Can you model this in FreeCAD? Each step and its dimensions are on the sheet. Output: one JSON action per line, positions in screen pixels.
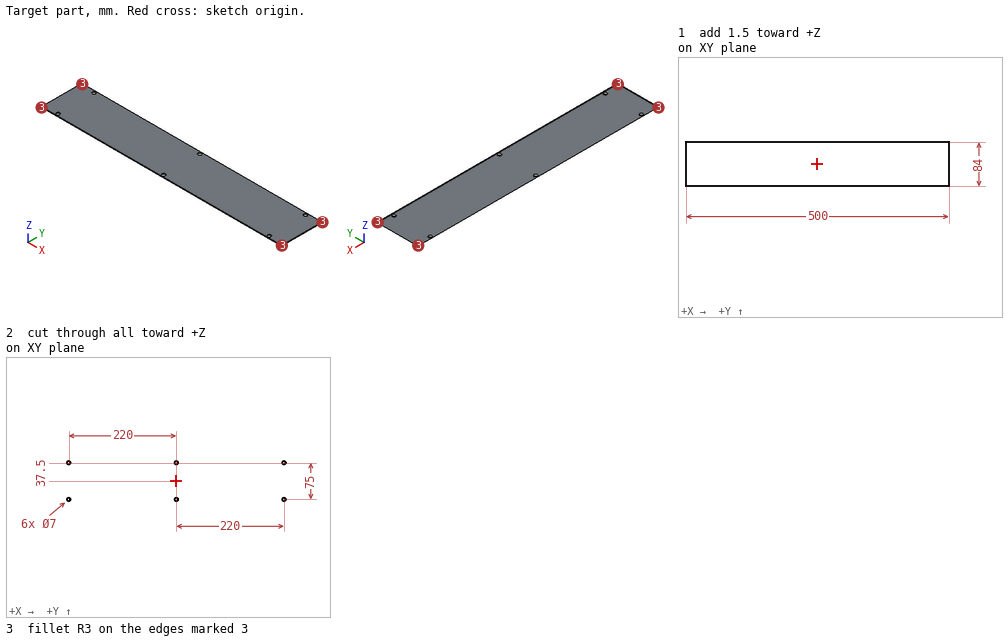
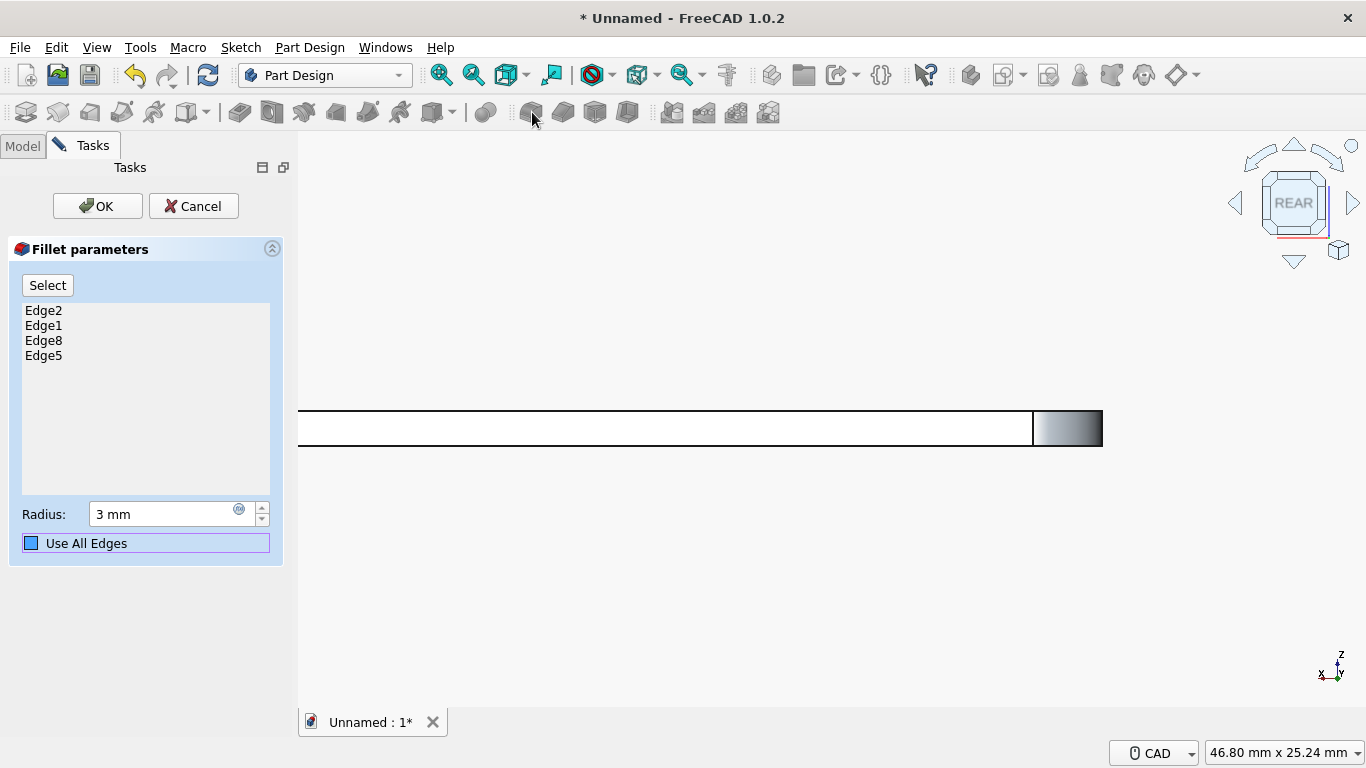
{"action": "left_click", "coordinate": [98, 206]}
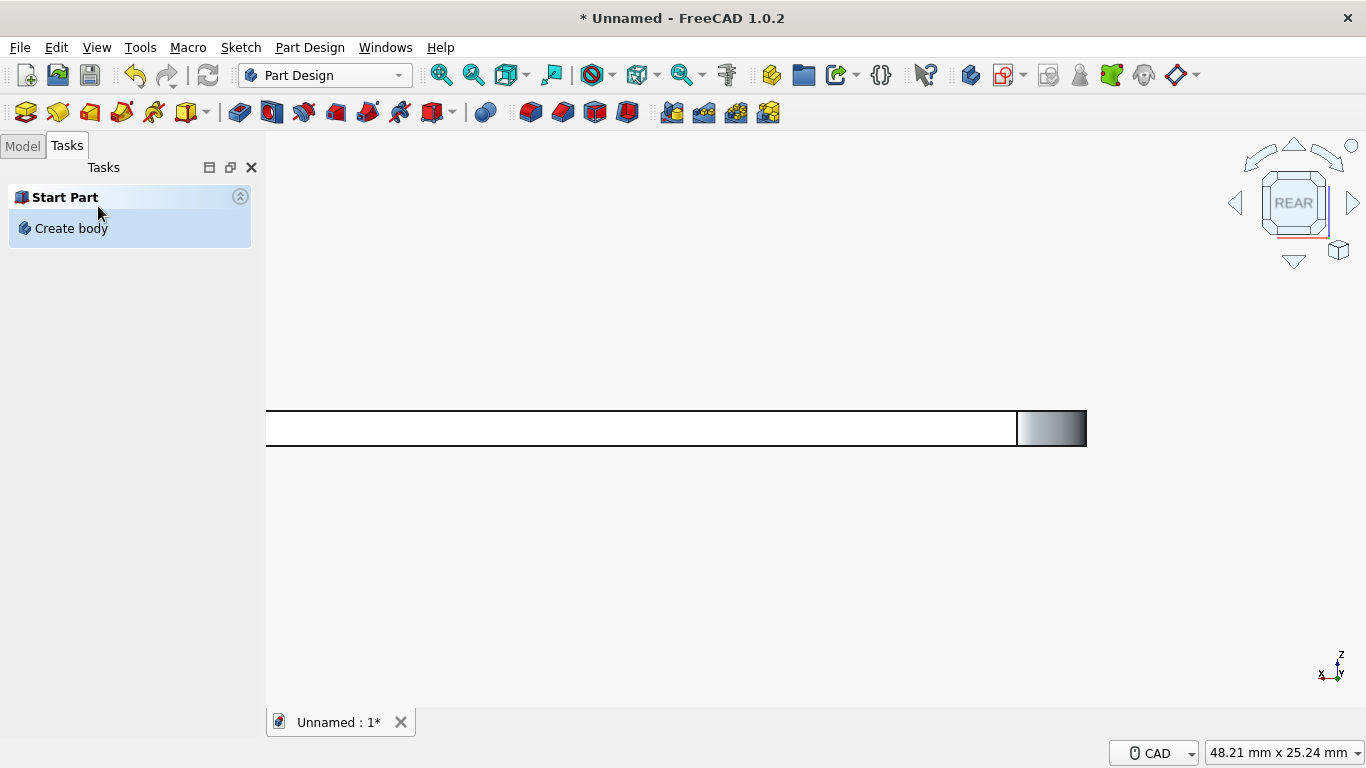
{"action": "key", "text": "0"}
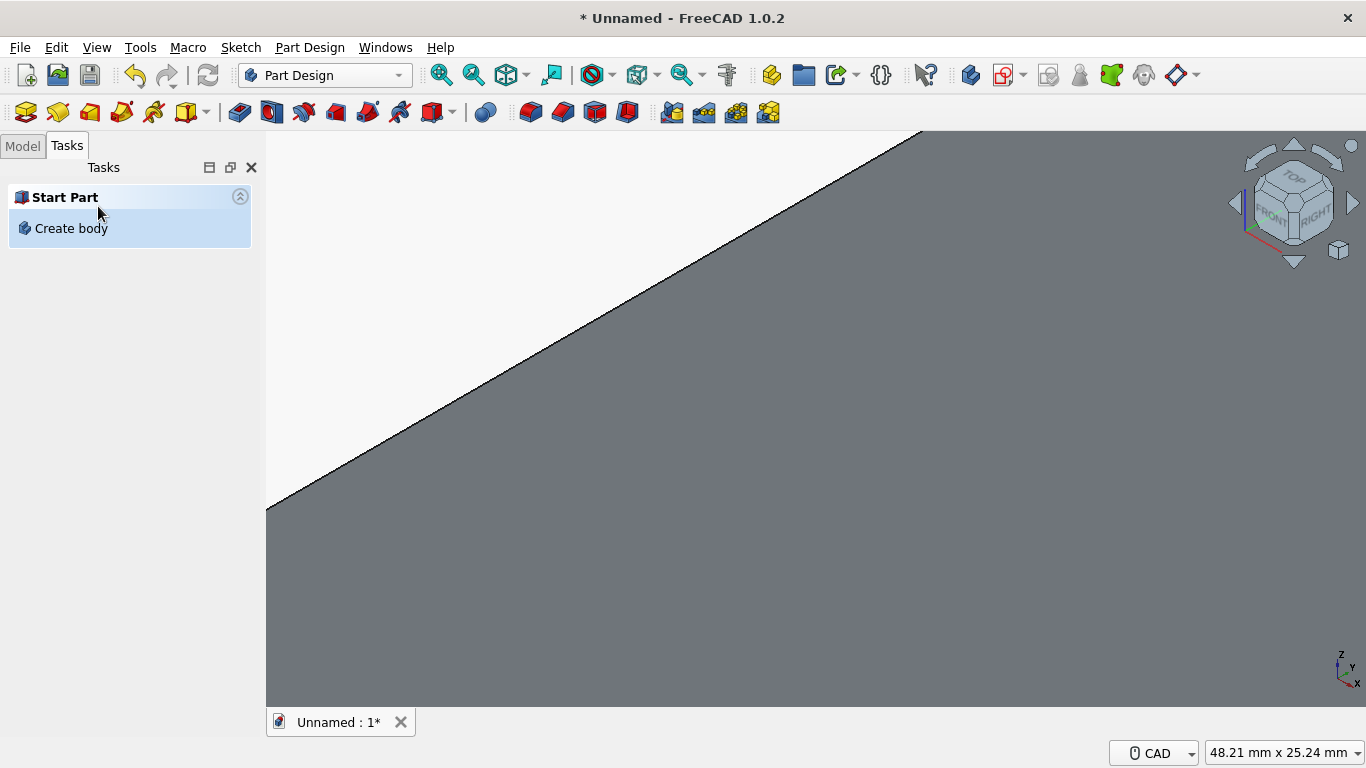
{"action": "left_click", "coordinate": [442, 76]}